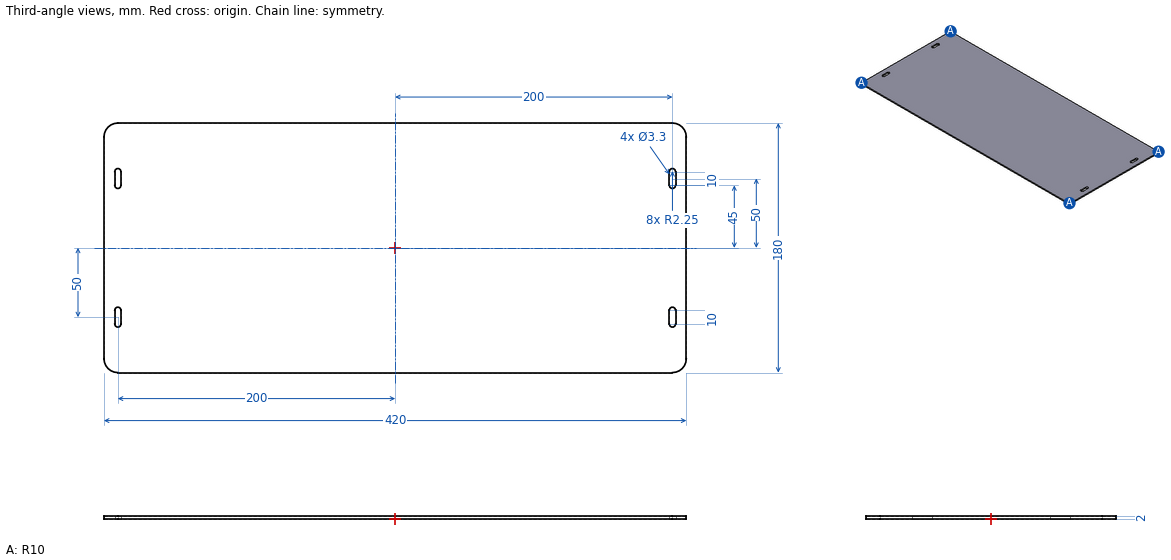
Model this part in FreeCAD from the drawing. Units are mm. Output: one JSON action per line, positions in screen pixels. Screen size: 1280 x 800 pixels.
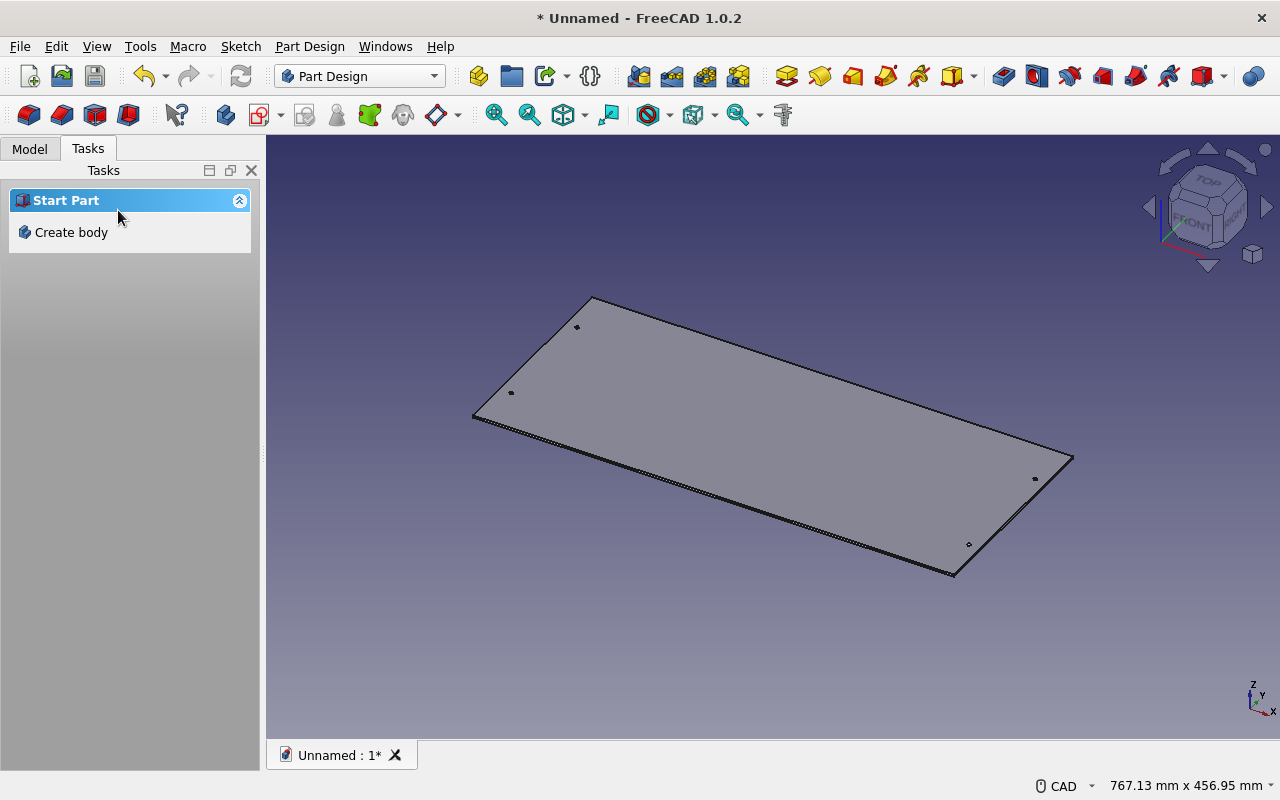
{"action": "left_click", "coordinate": [910, 480]}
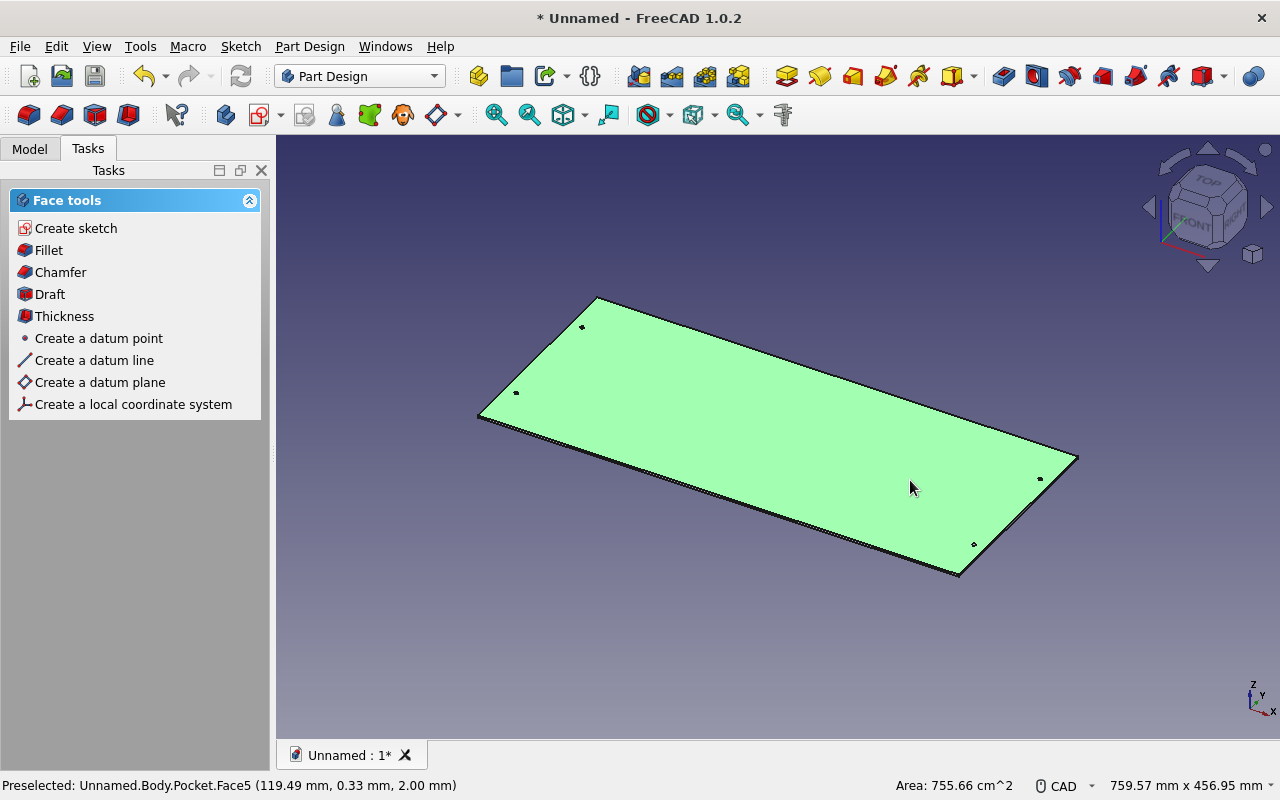
{"action": "left_click", "coordinate": [258, 116]}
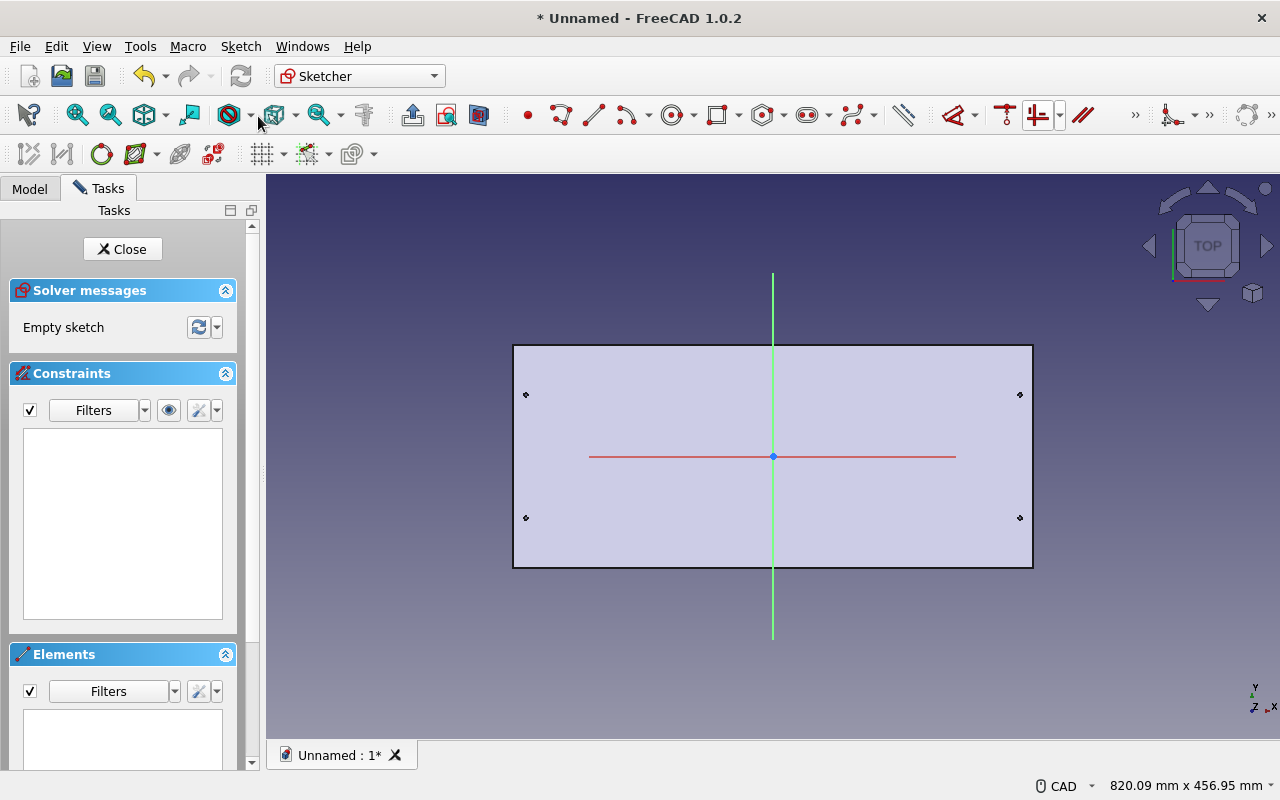
{"action": "key", "text": "g s"}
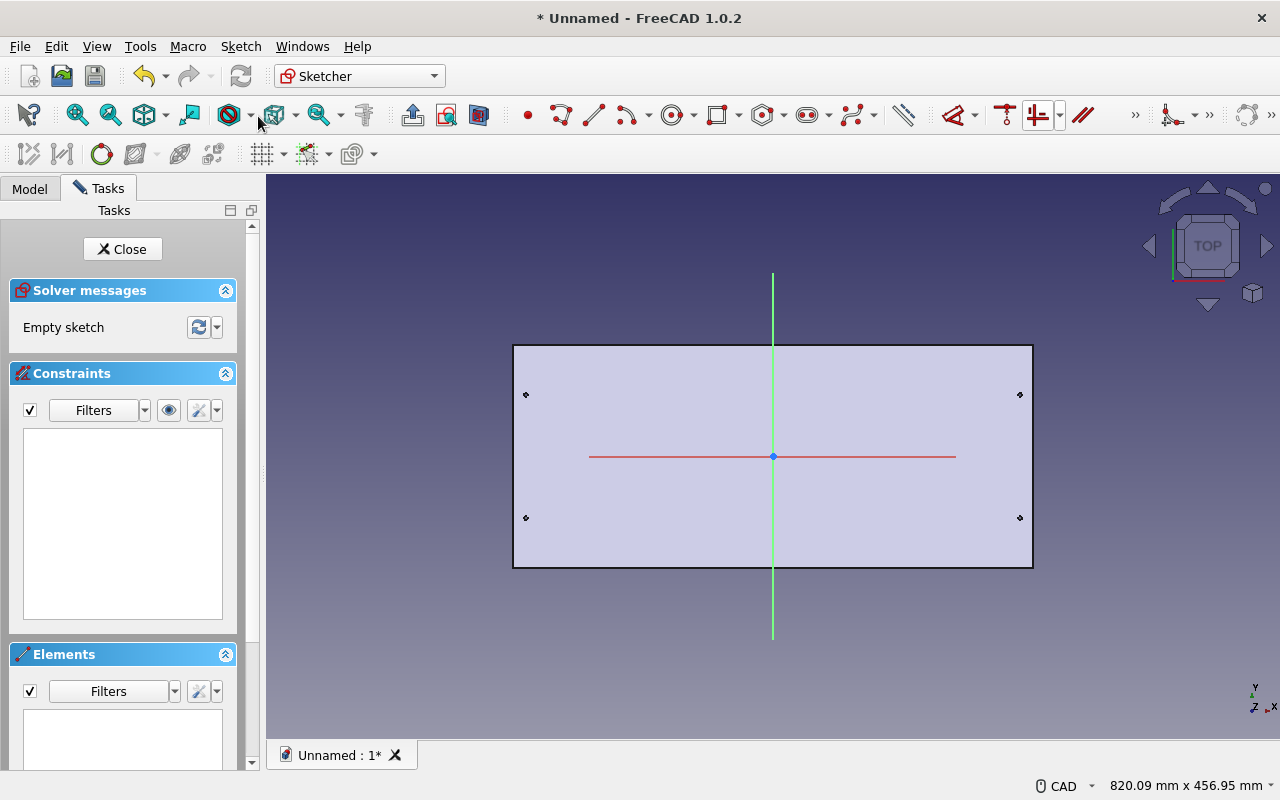
{"action": "scroll", "coordinate": [1020, 401], "scroll_direction": "up", "scroll_amount": 11}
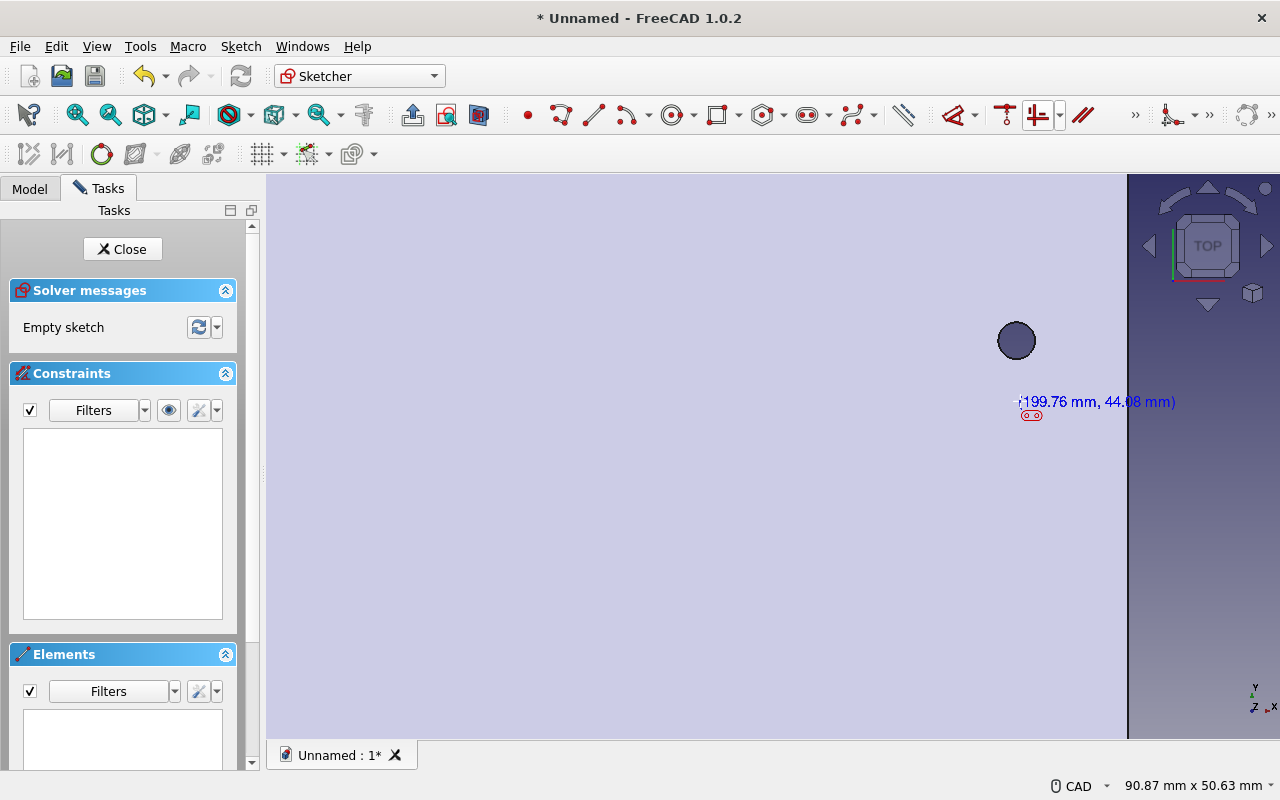
{"action": "scroll", "coordinate": [1005, 387], "scroll_direction": "down", "scroll_amount": 10}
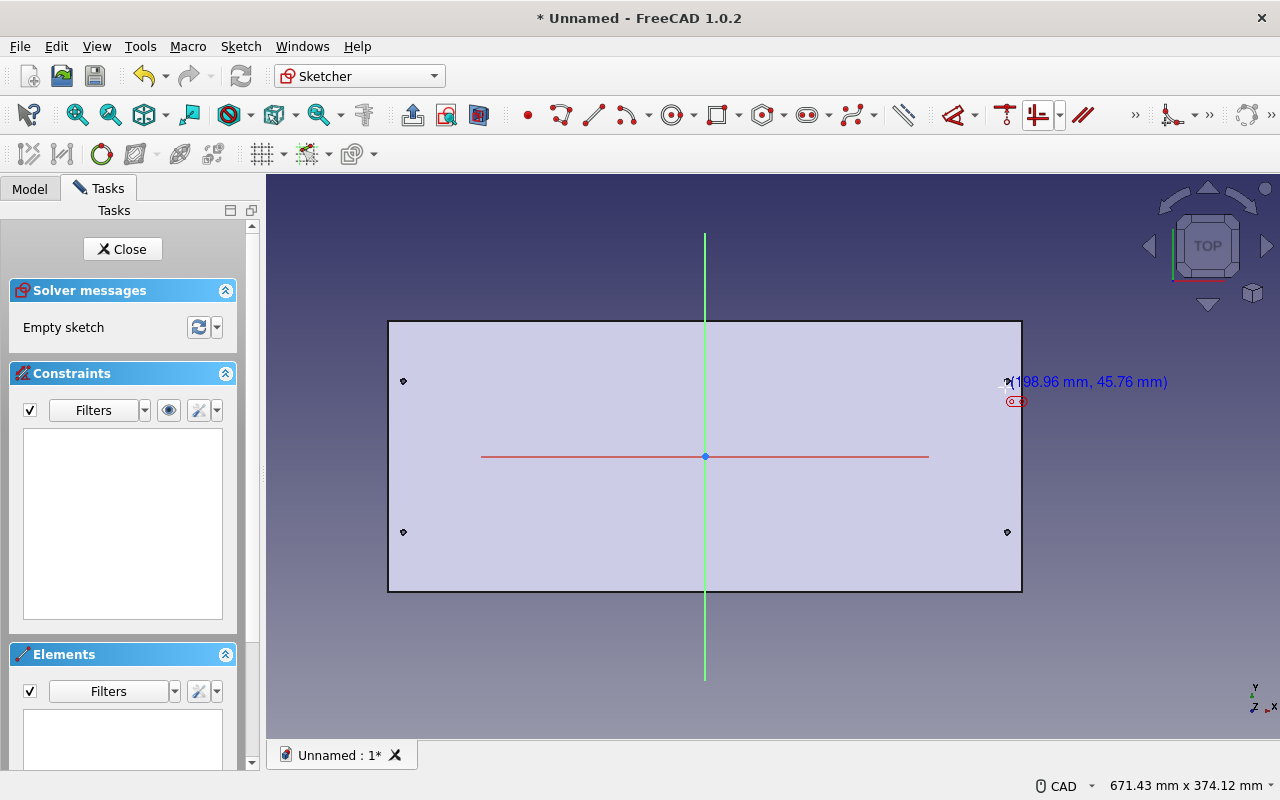
{"action": "left_click", "coordinate": [1007, 389]}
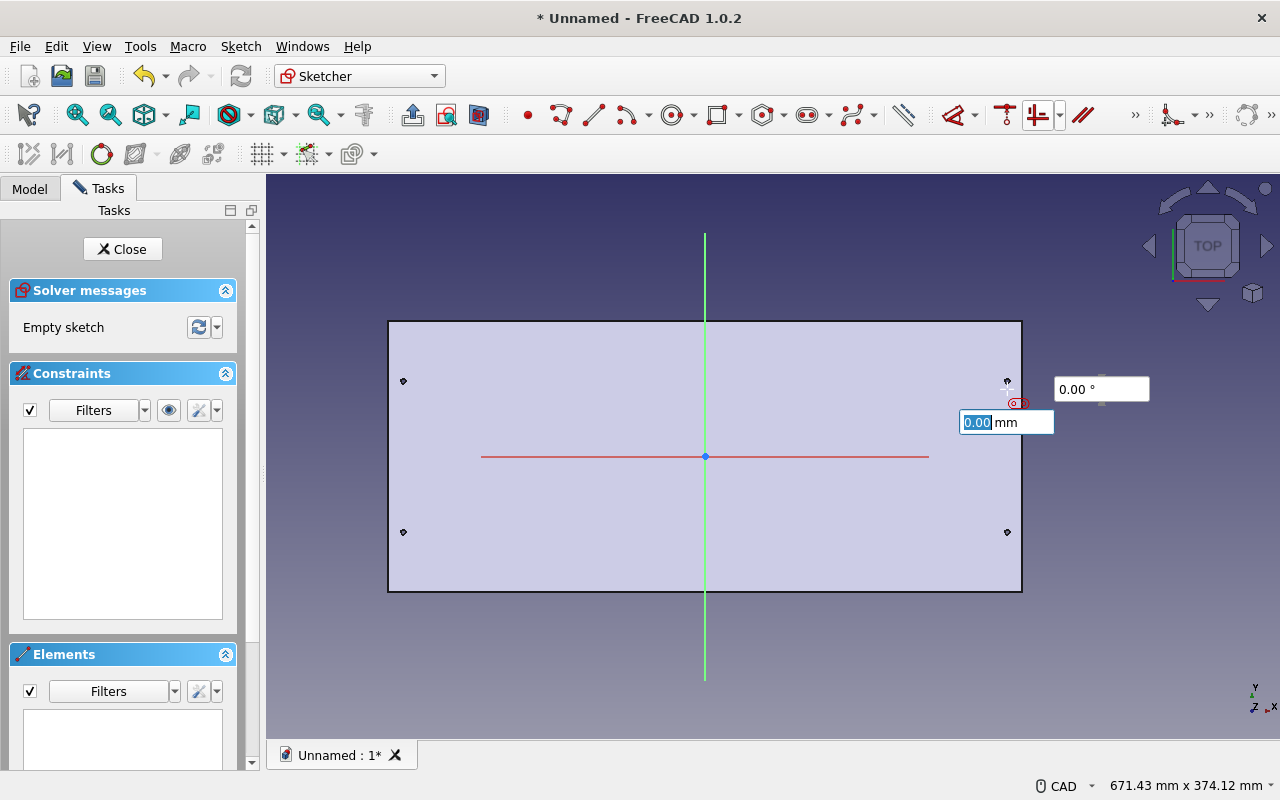
{"action": "left_click", "coordinate": [1007, 374]}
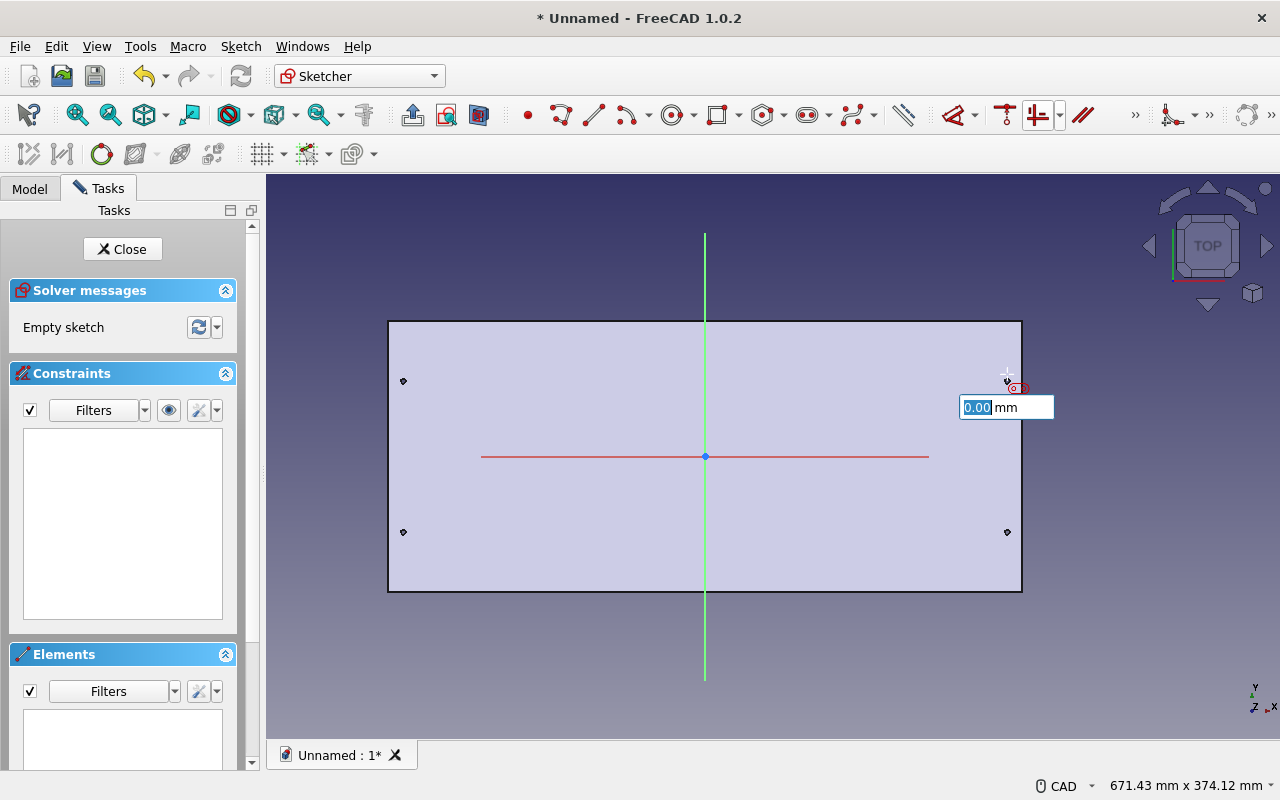
{"action": "scroll", "coordinate": [1011, 381], "scroll_direction": "up", "scroll_amount": 8}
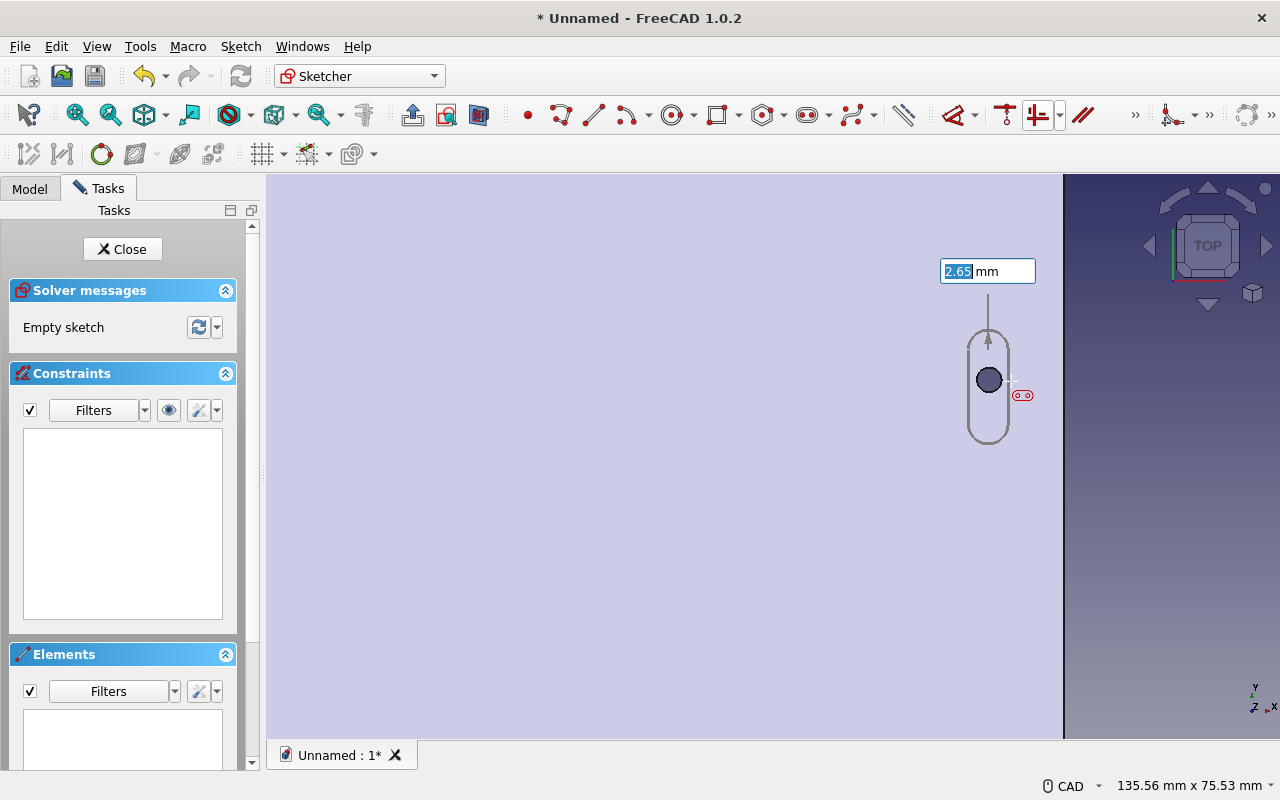
{"action": "left_click", "coordinate": [1006, 380]}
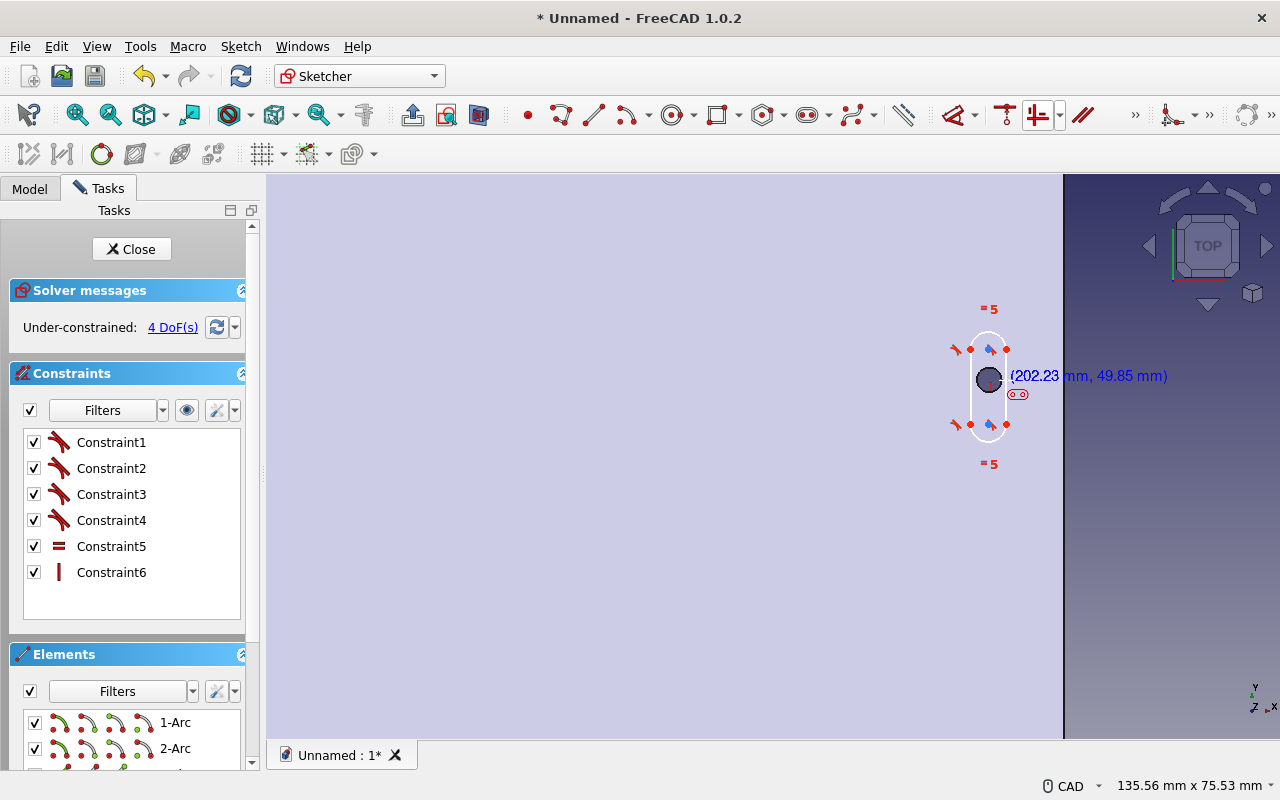
{"action": "scroll", "coordinate": [1011, 381], "scroll_direction": "down", "scroll_amount": 8}